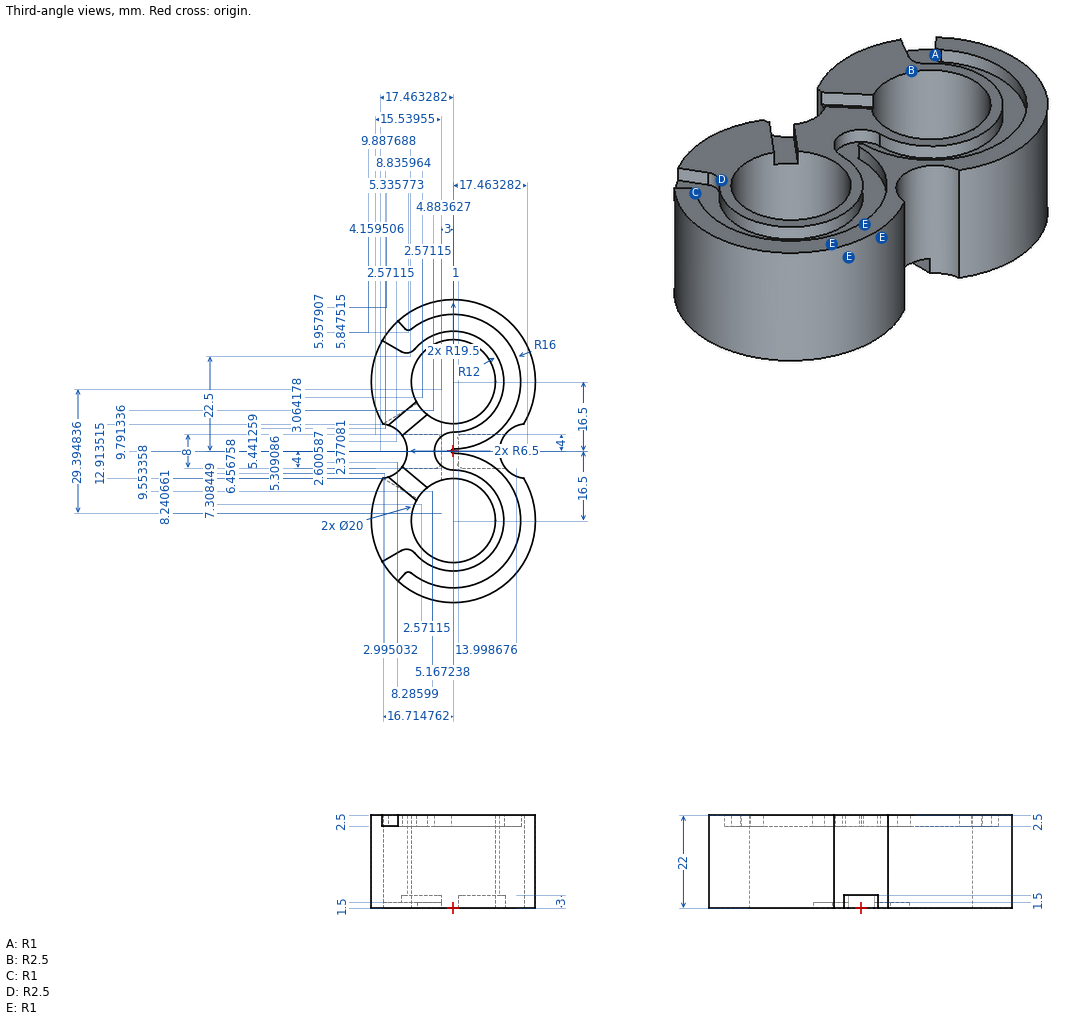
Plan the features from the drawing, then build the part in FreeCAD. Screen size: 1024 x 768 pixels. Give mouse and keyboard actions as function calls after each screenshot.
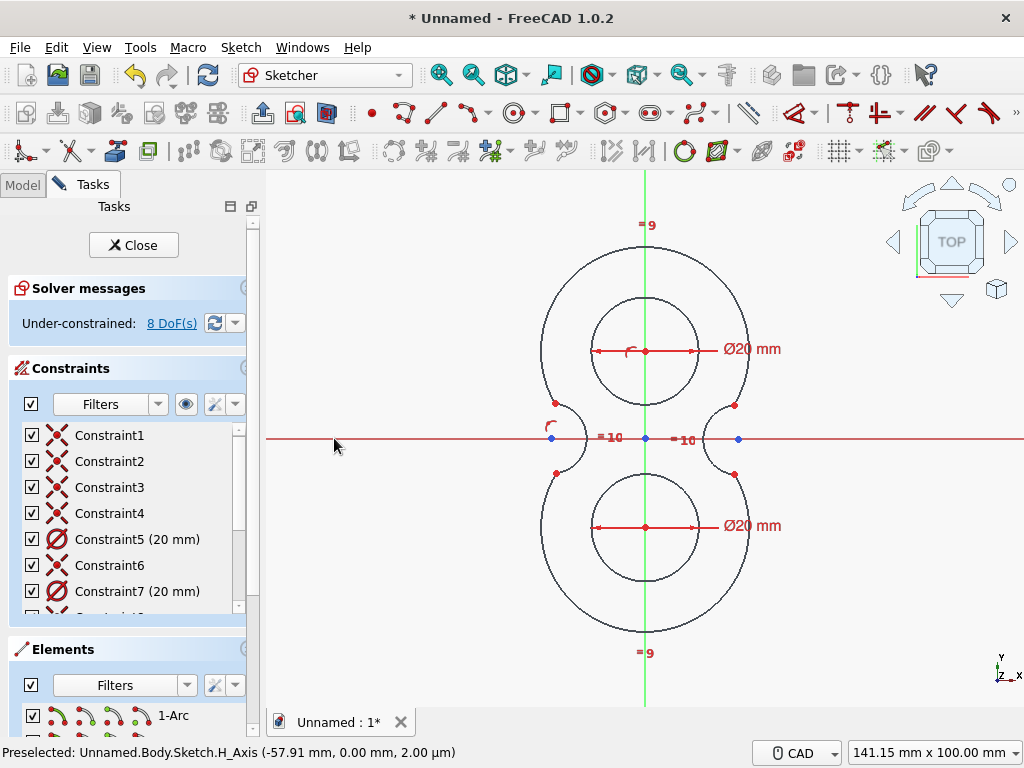
click(645, 528)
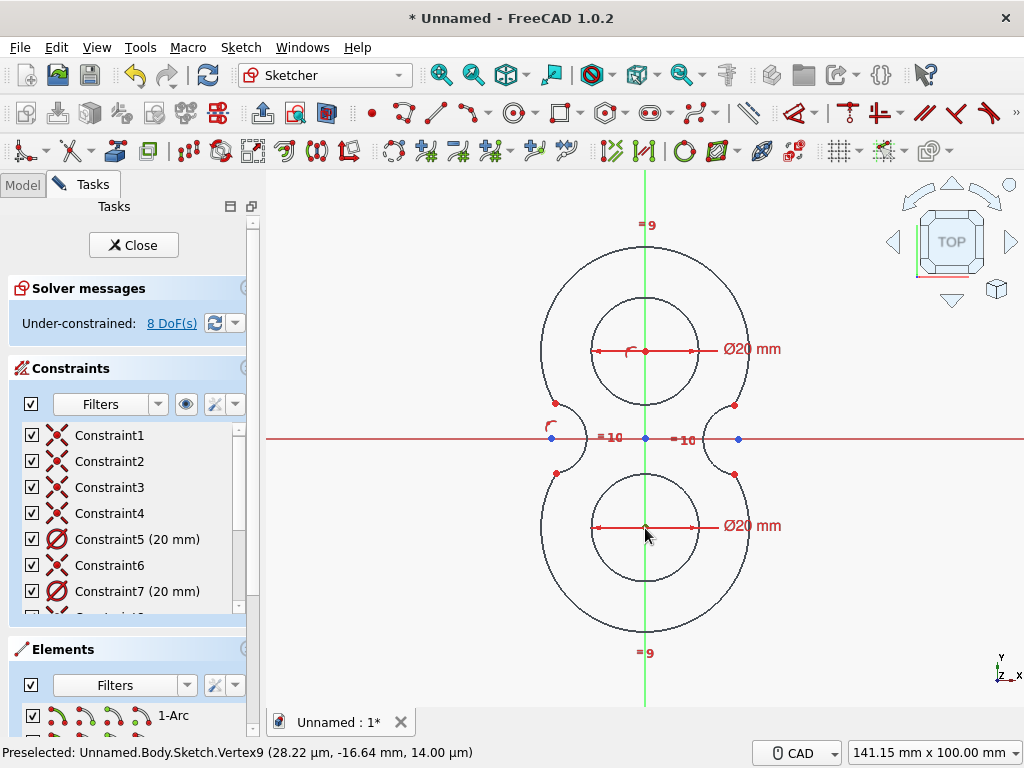
click(645, 542)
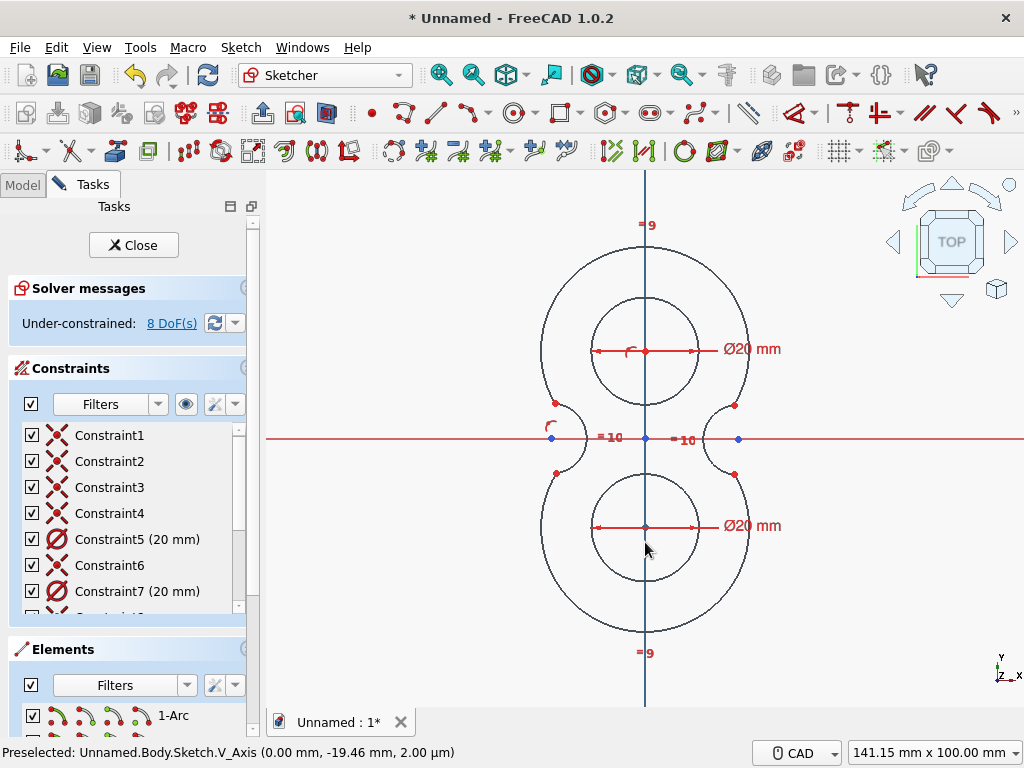
click(848, 114)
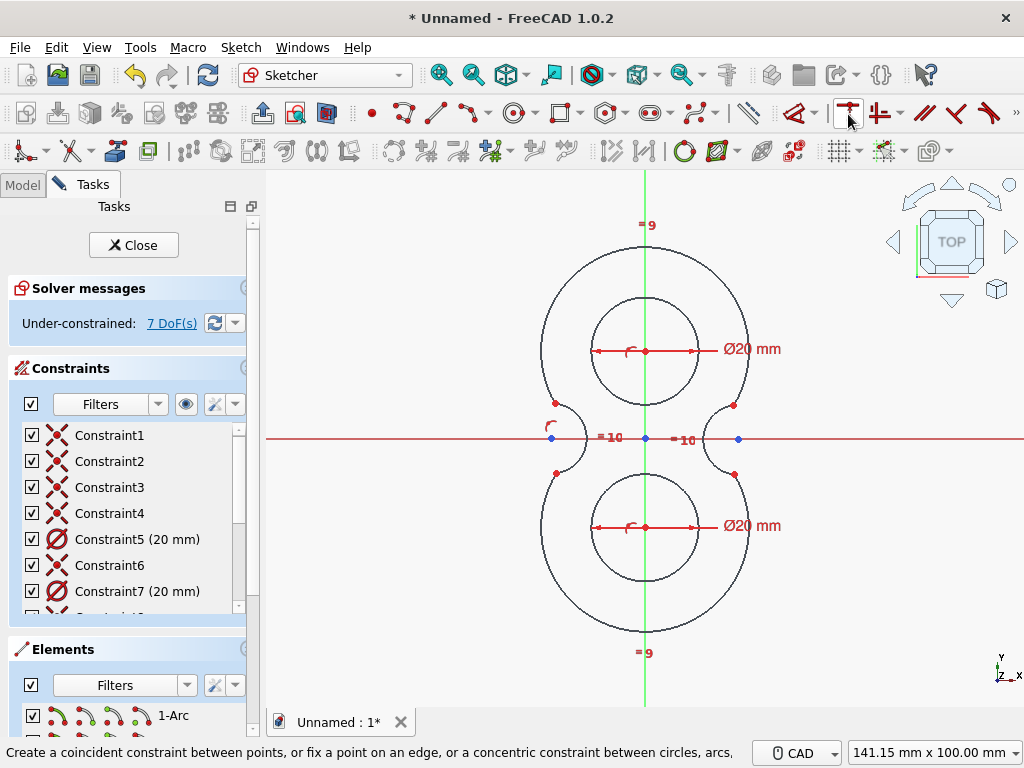
click(738, 440)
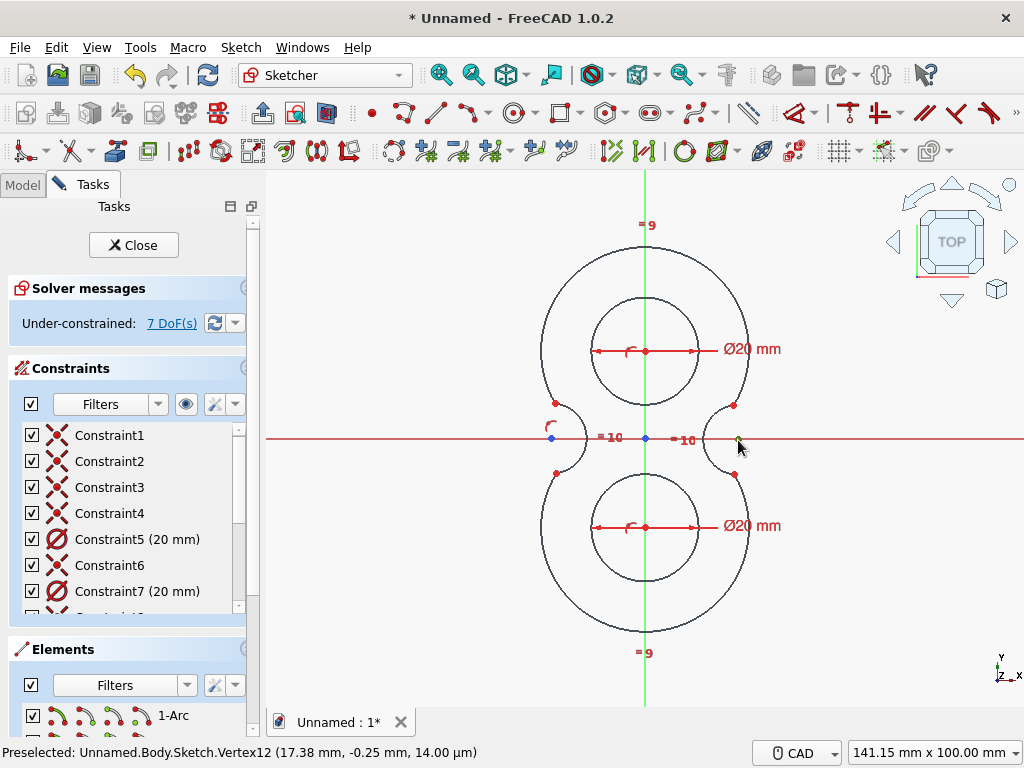
click(334, 438)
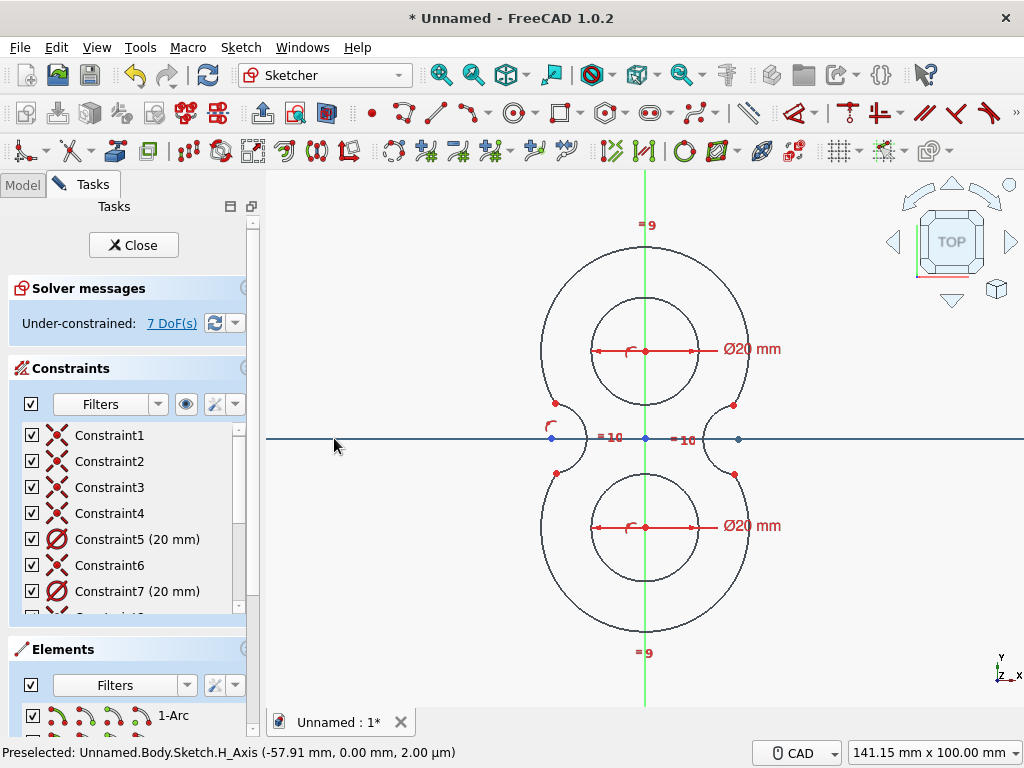
key(c)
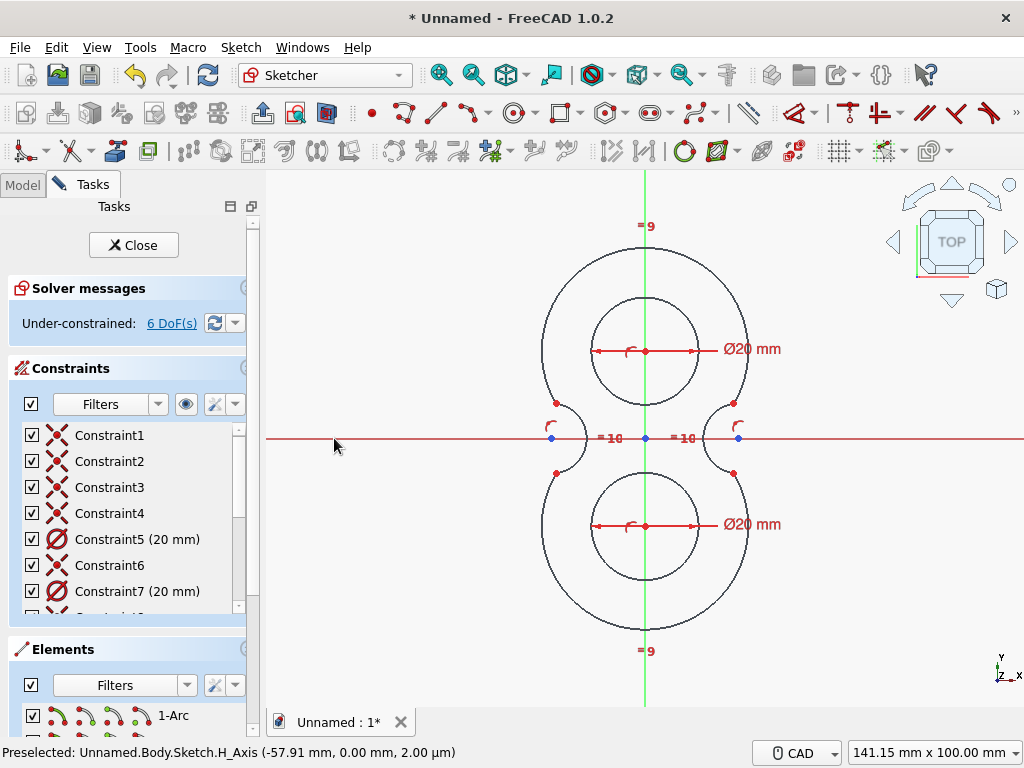
click(722, 282)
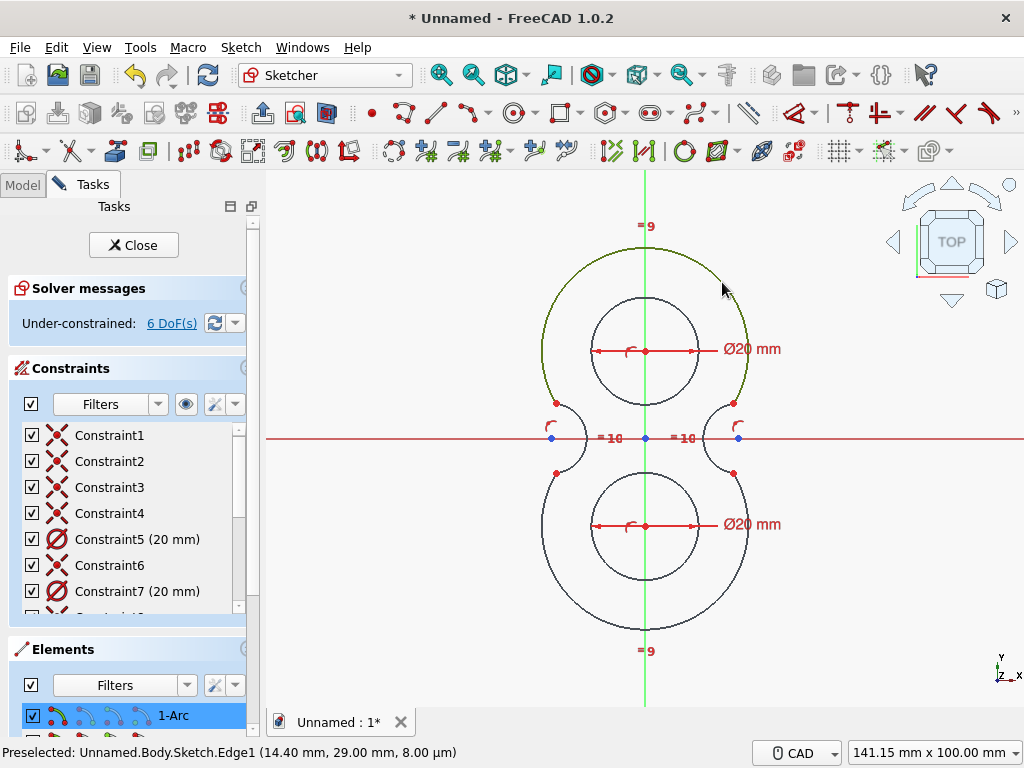
key(k)
key(r)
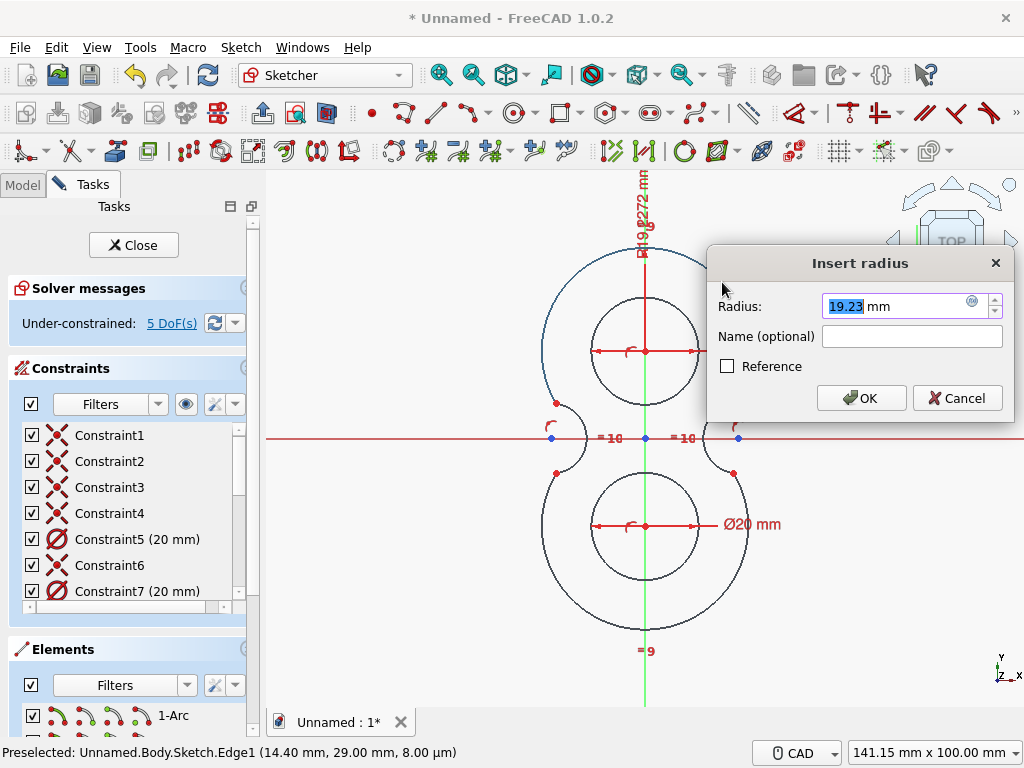
text(19.5)
key(Return)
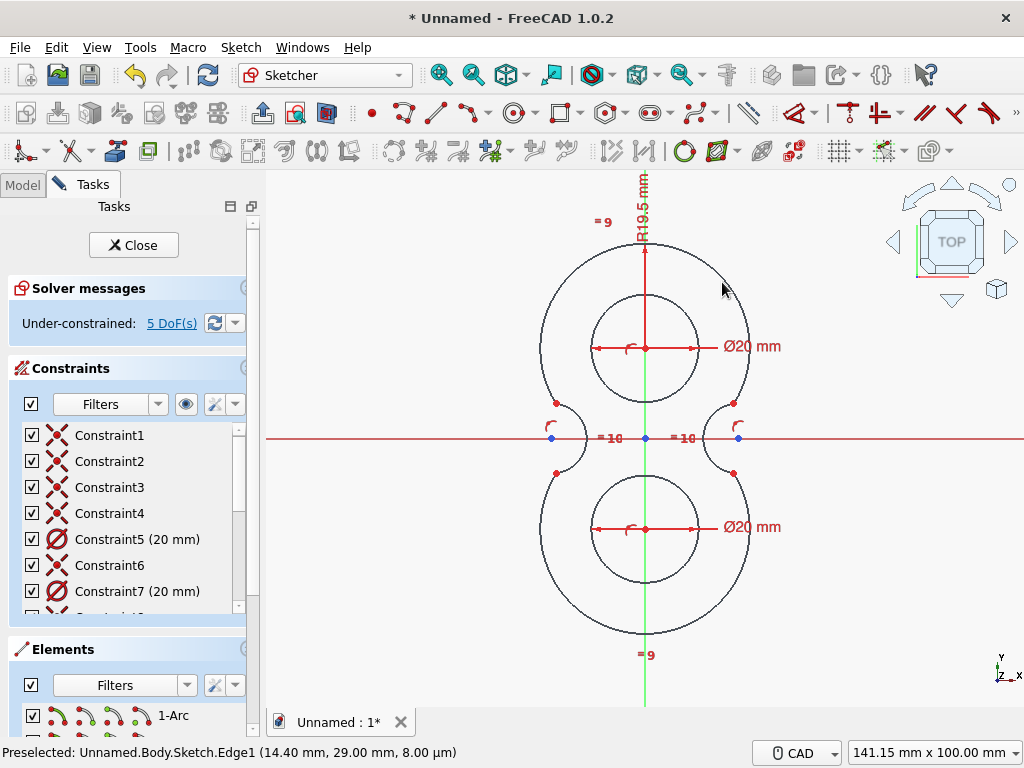
click(581, 457)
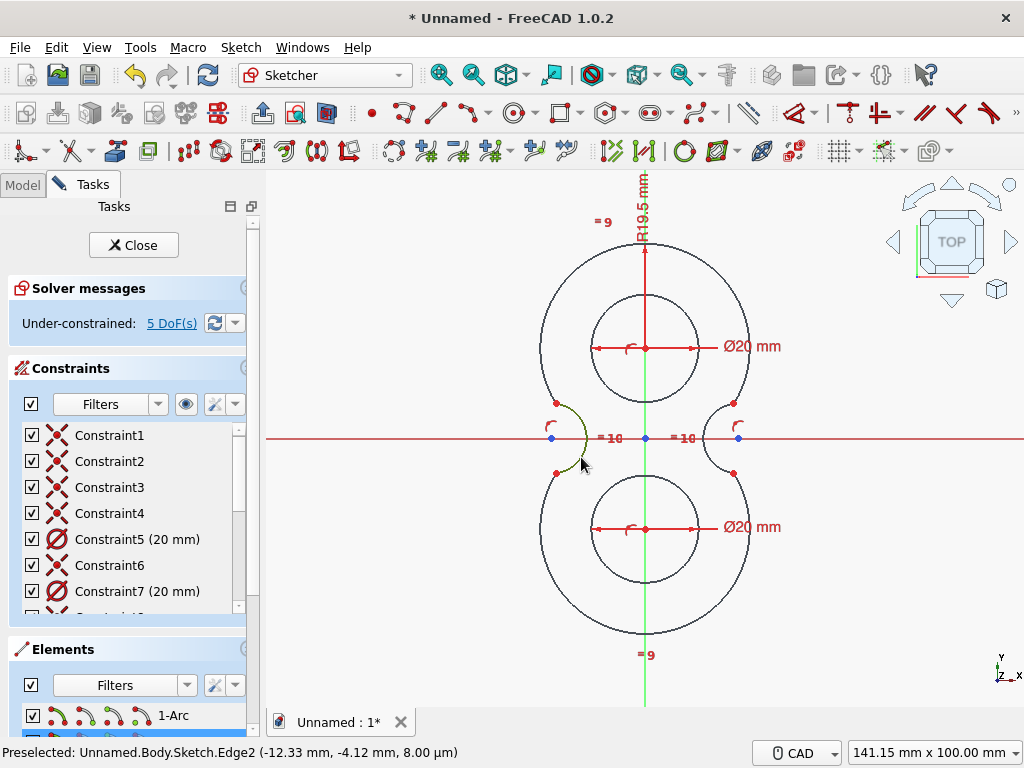
key(k)
key(r)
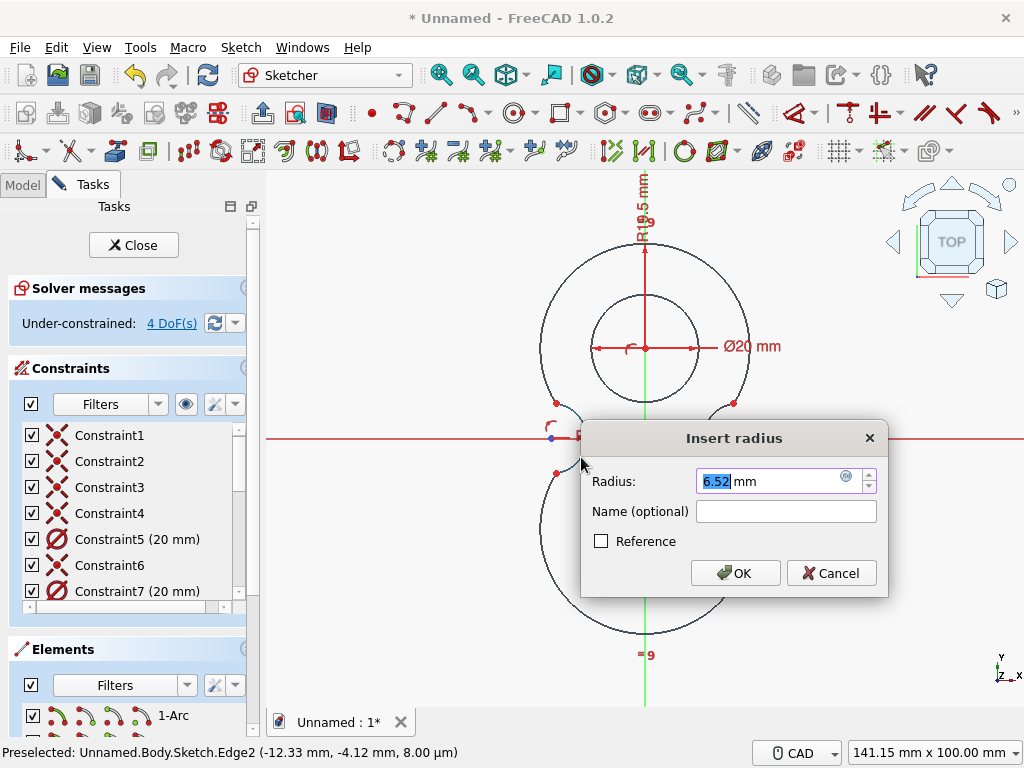
text(6.5)
key(Return)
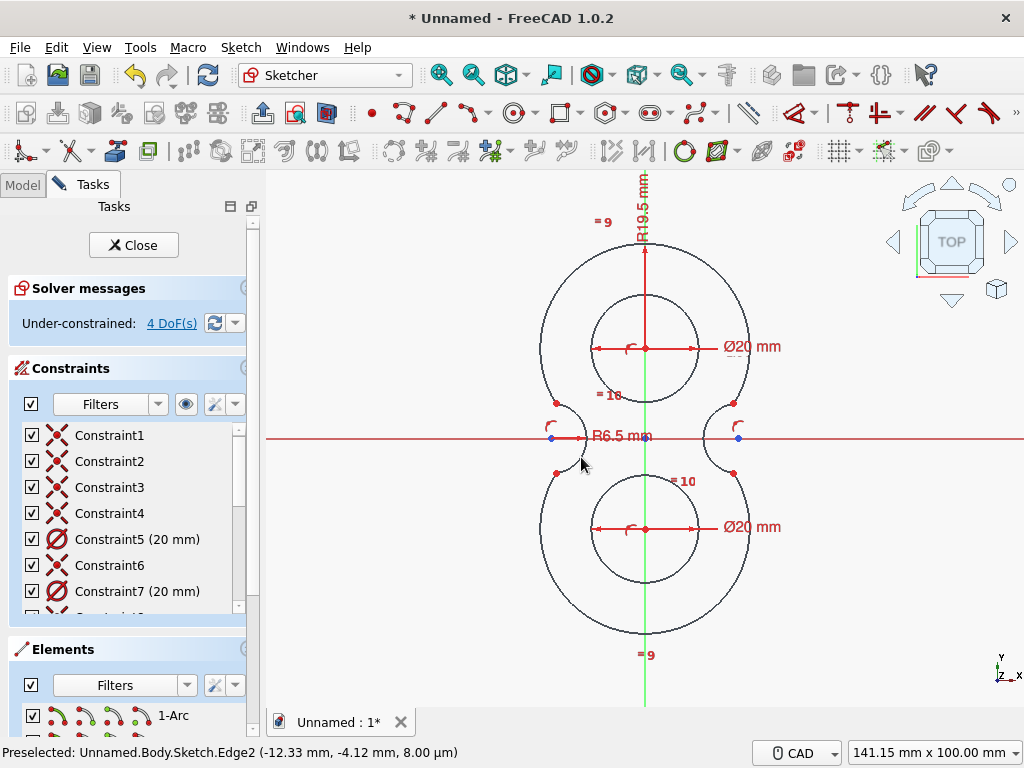
click(645, 529)